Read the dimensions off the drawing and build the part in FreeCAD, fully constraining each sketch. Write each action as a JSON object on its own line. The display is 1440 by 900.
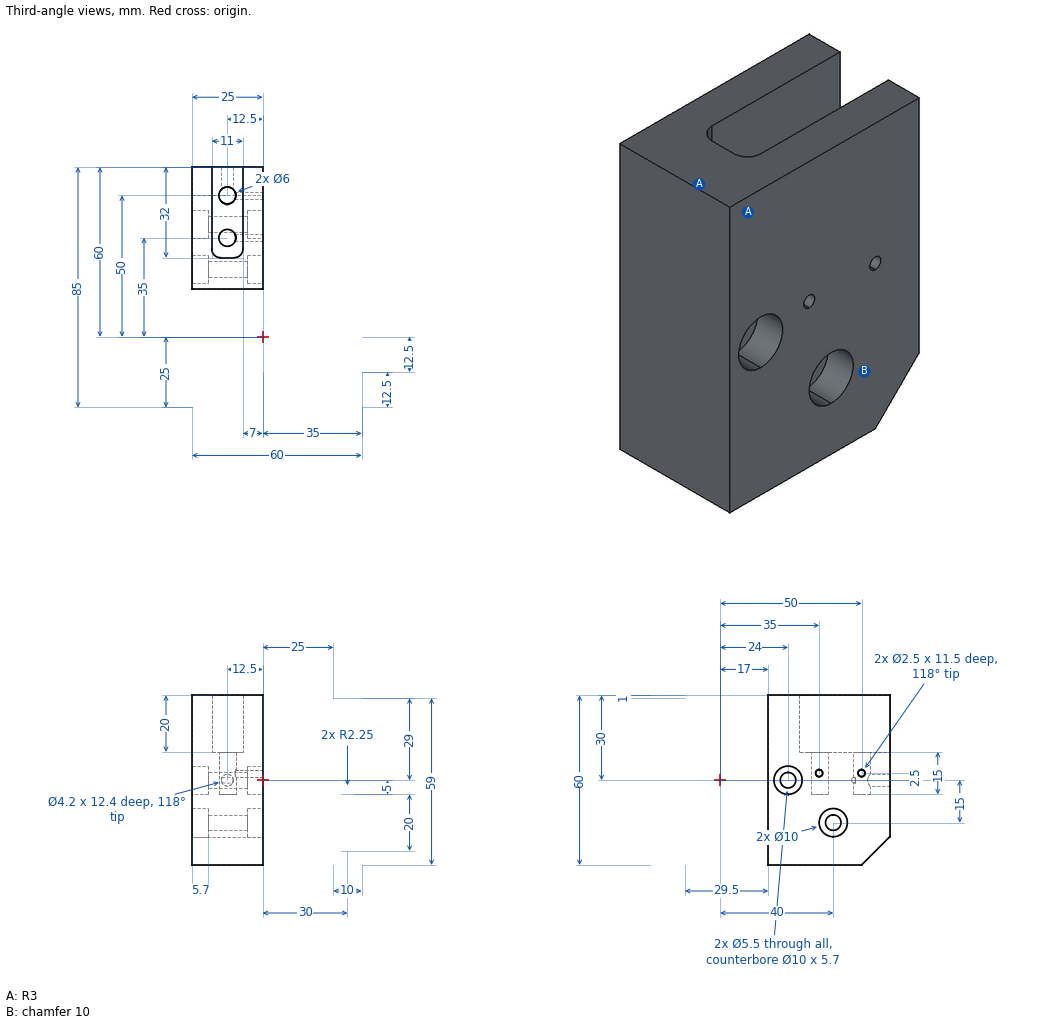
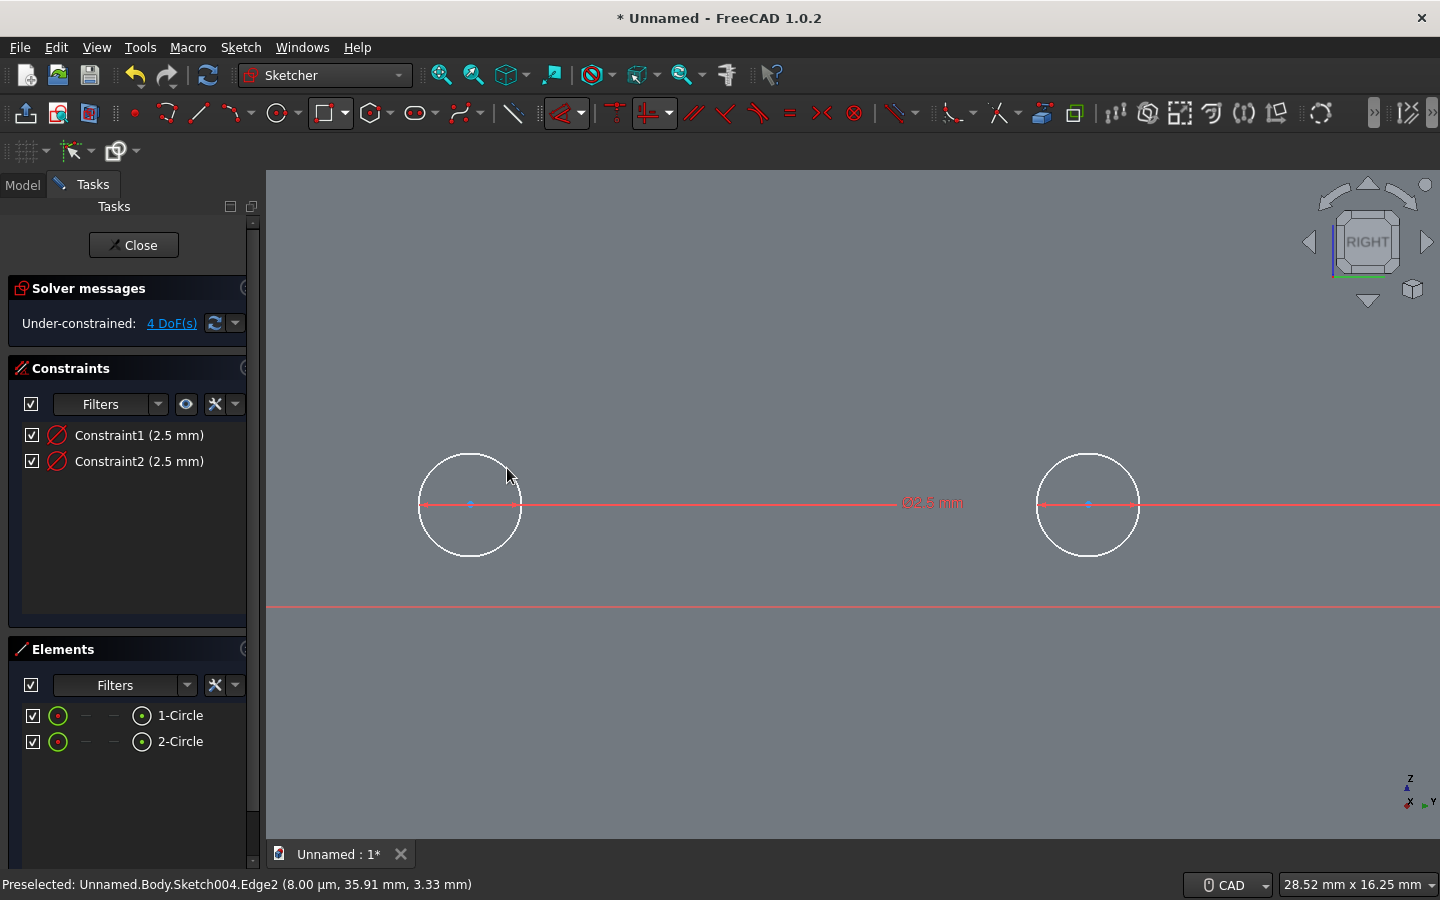
{"action": "left_click", "coordinate": [1088, 505]}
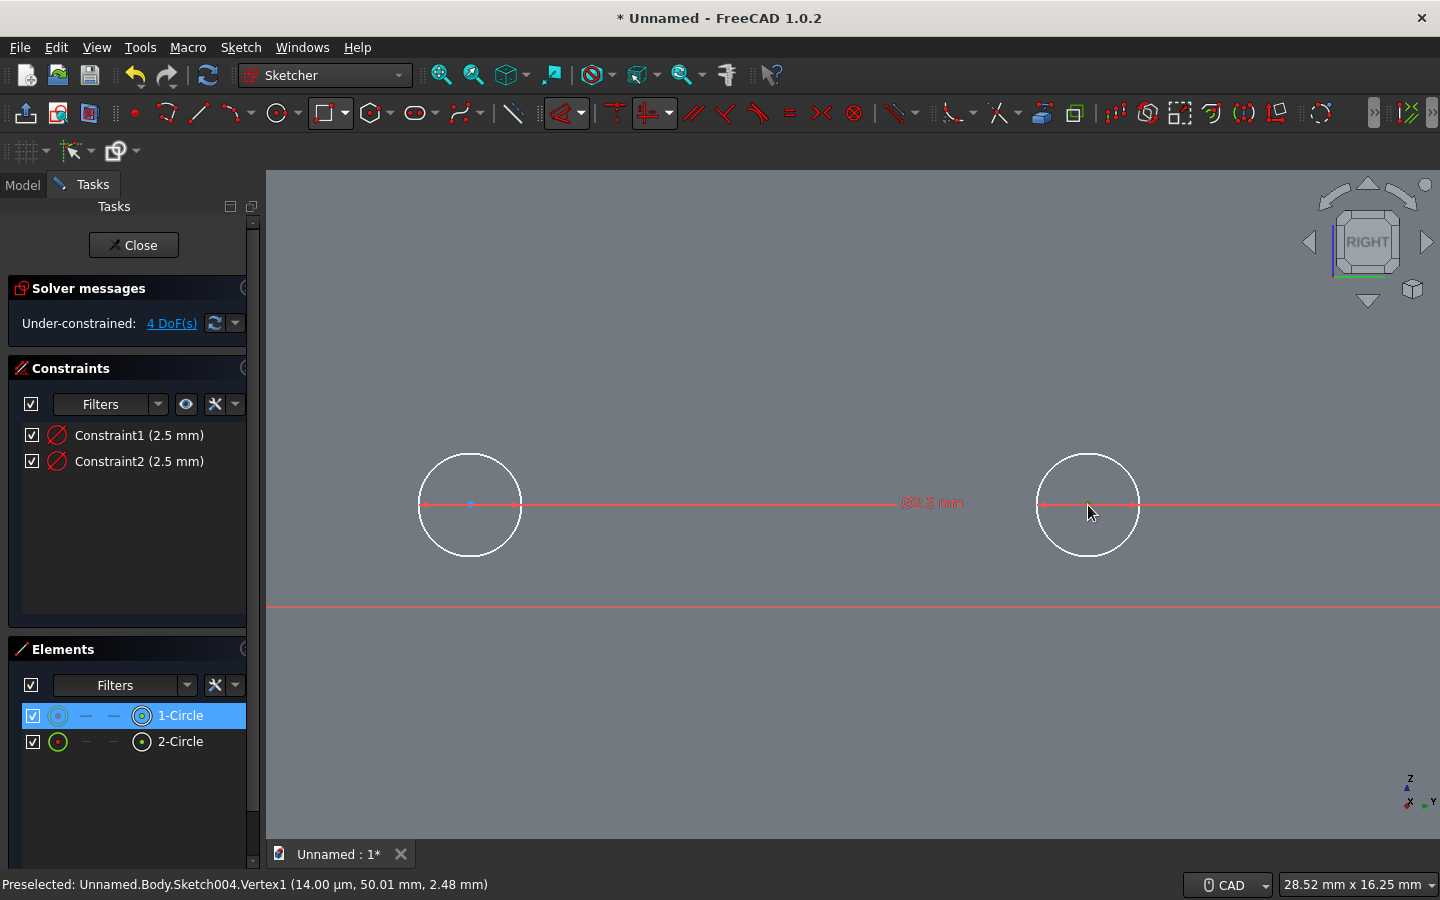
{"action": "left_click", "coordinate": [470, 505]}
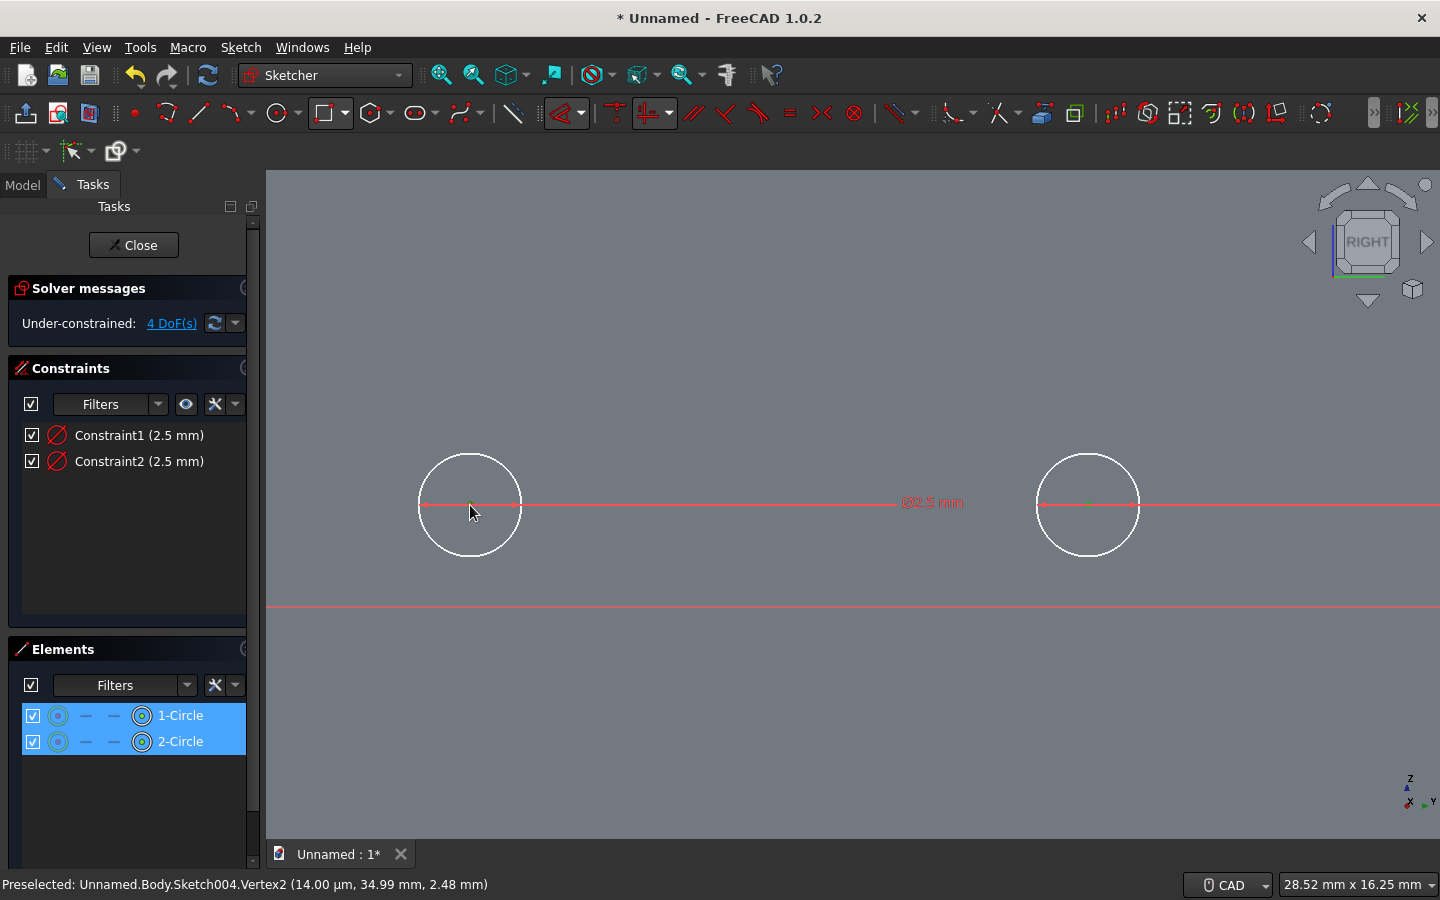
{"action": "key", "text": "h"}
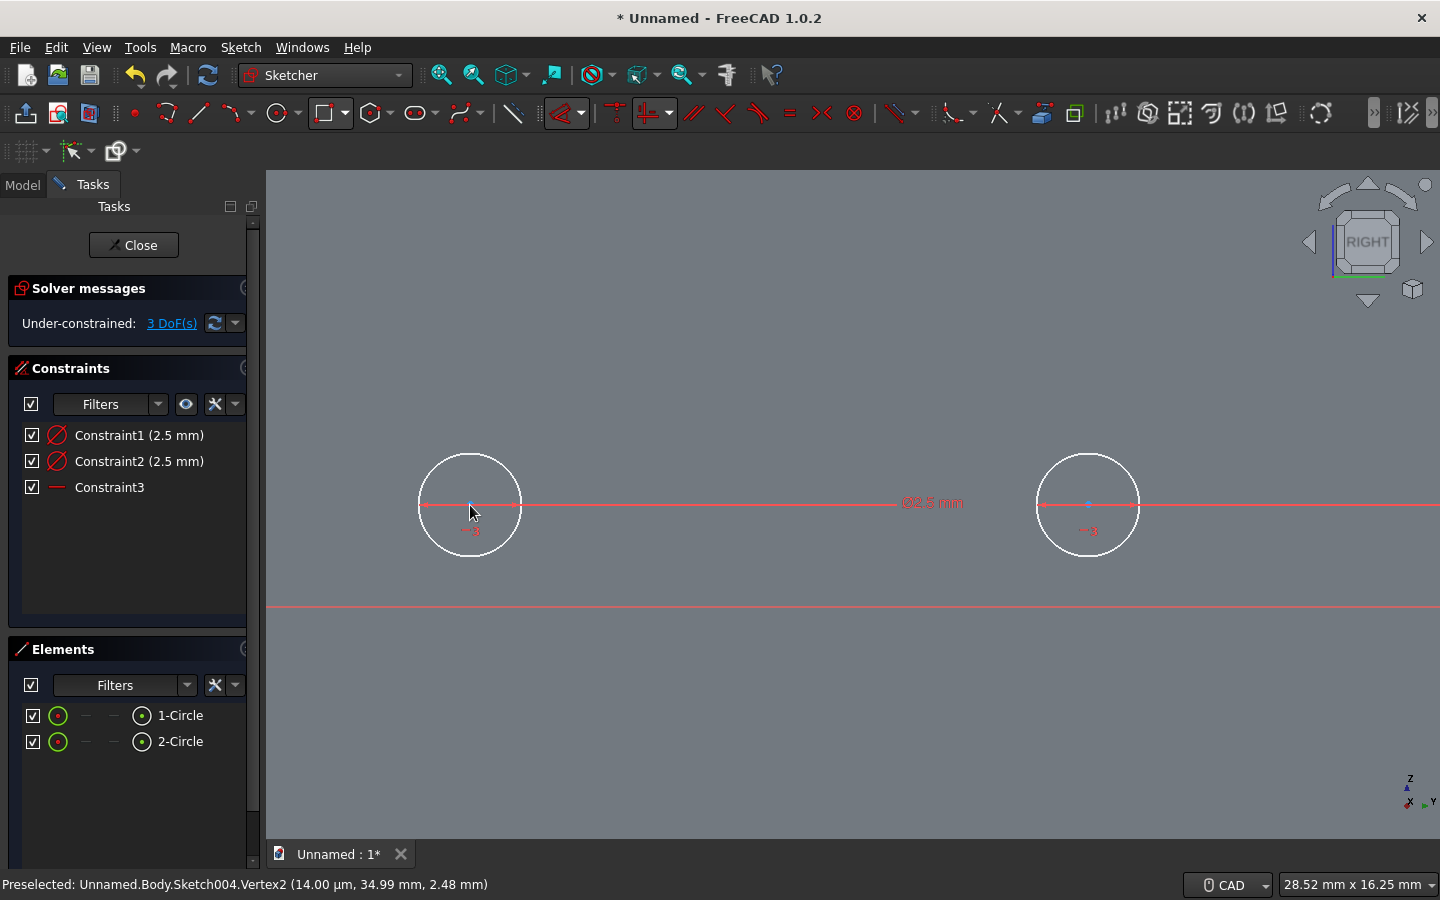
{"action": "left_click", "coordinate": [1088, 505]}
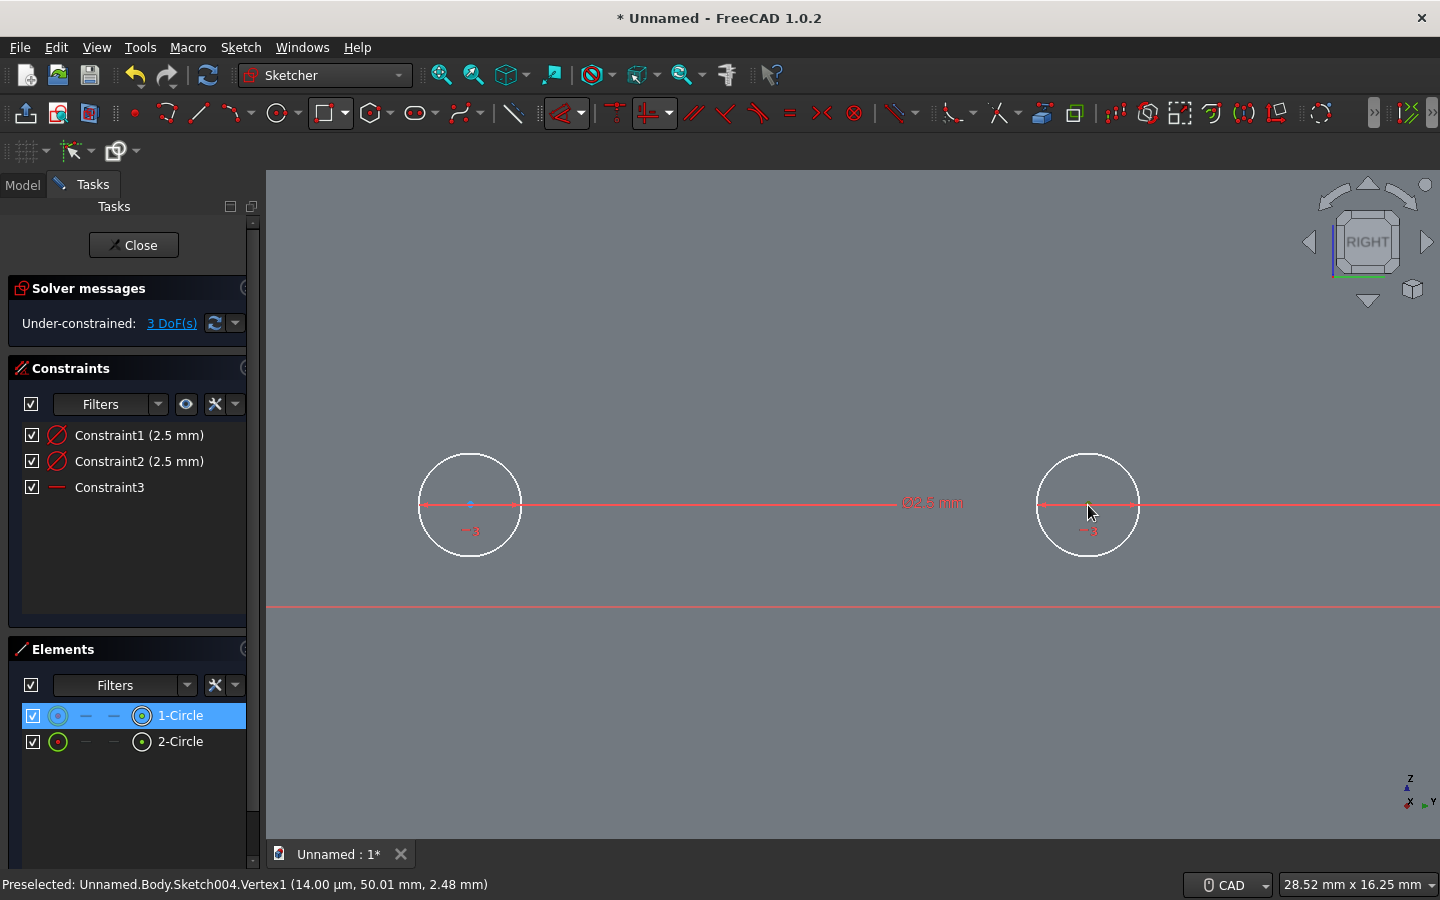
{"action": "key", "text": "l"}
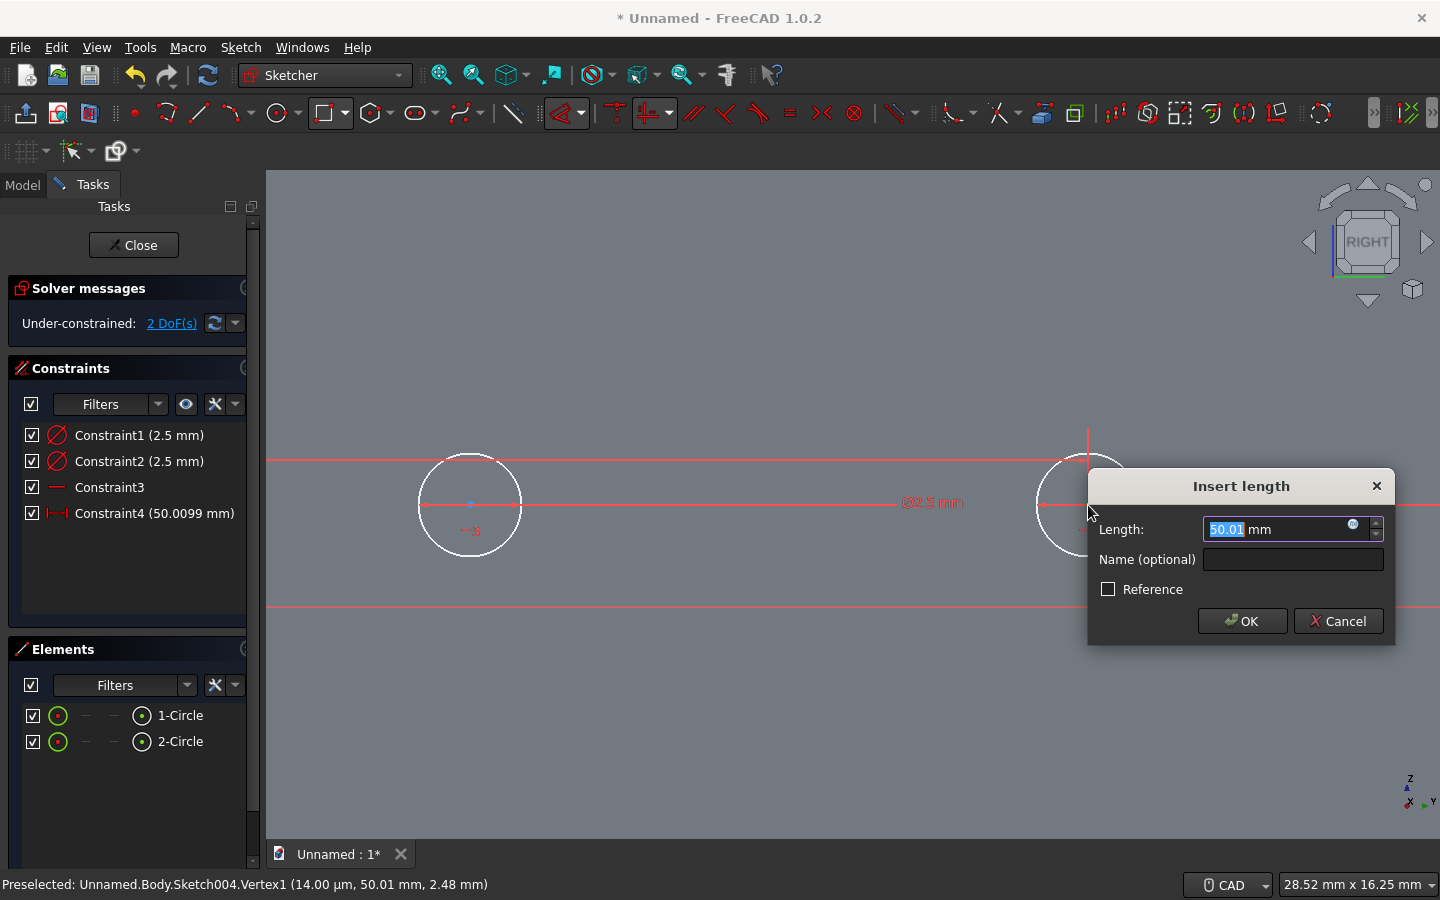
{"action": "type", "text": "50"}
{"action": "key", "text": "Return"}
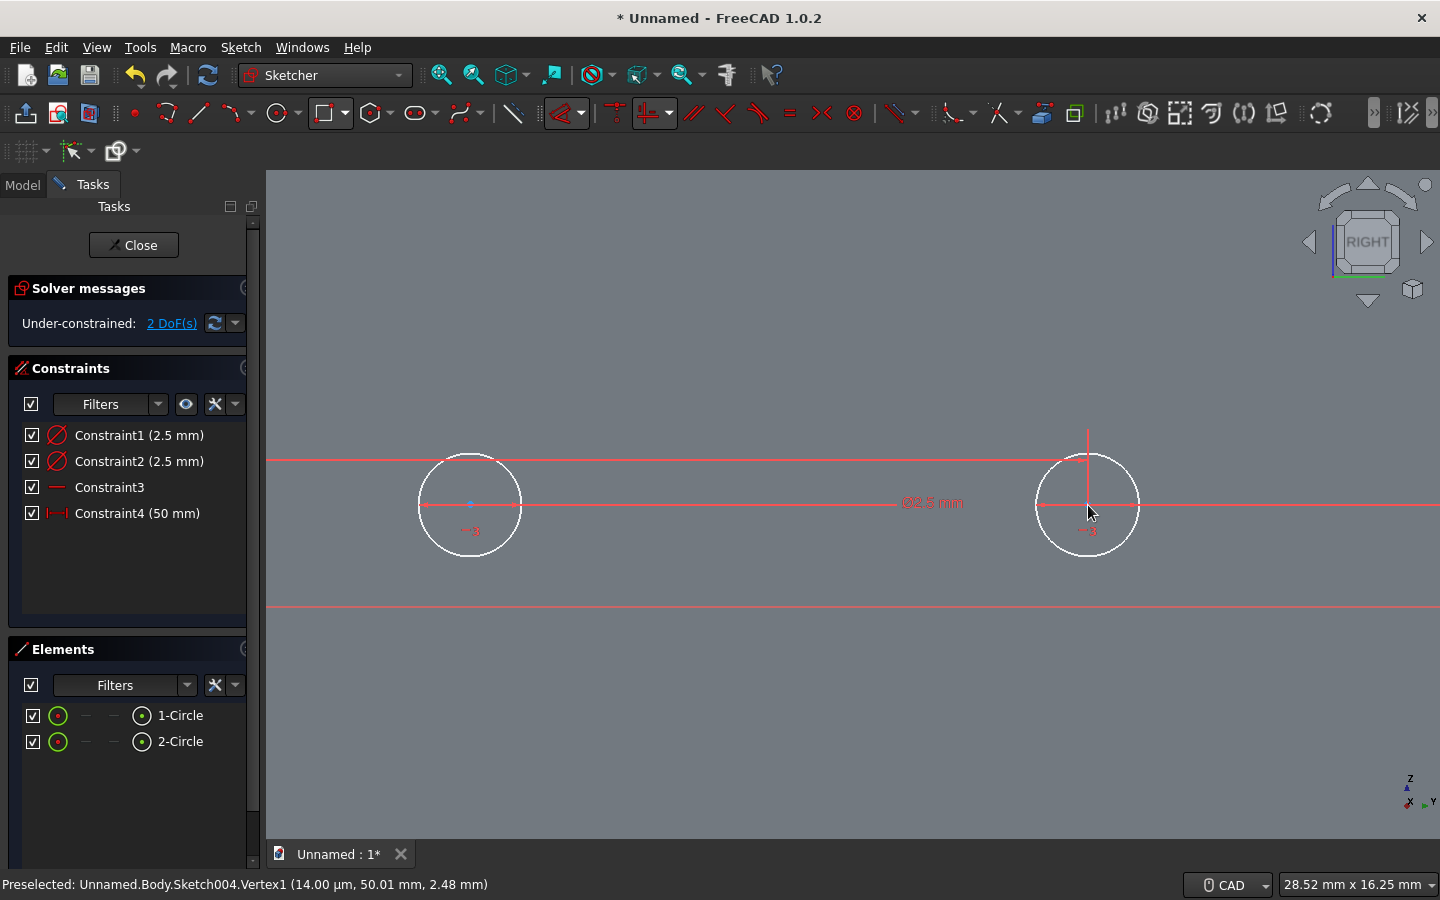
{"action": "left_click", "coordinate": [470, 505]}